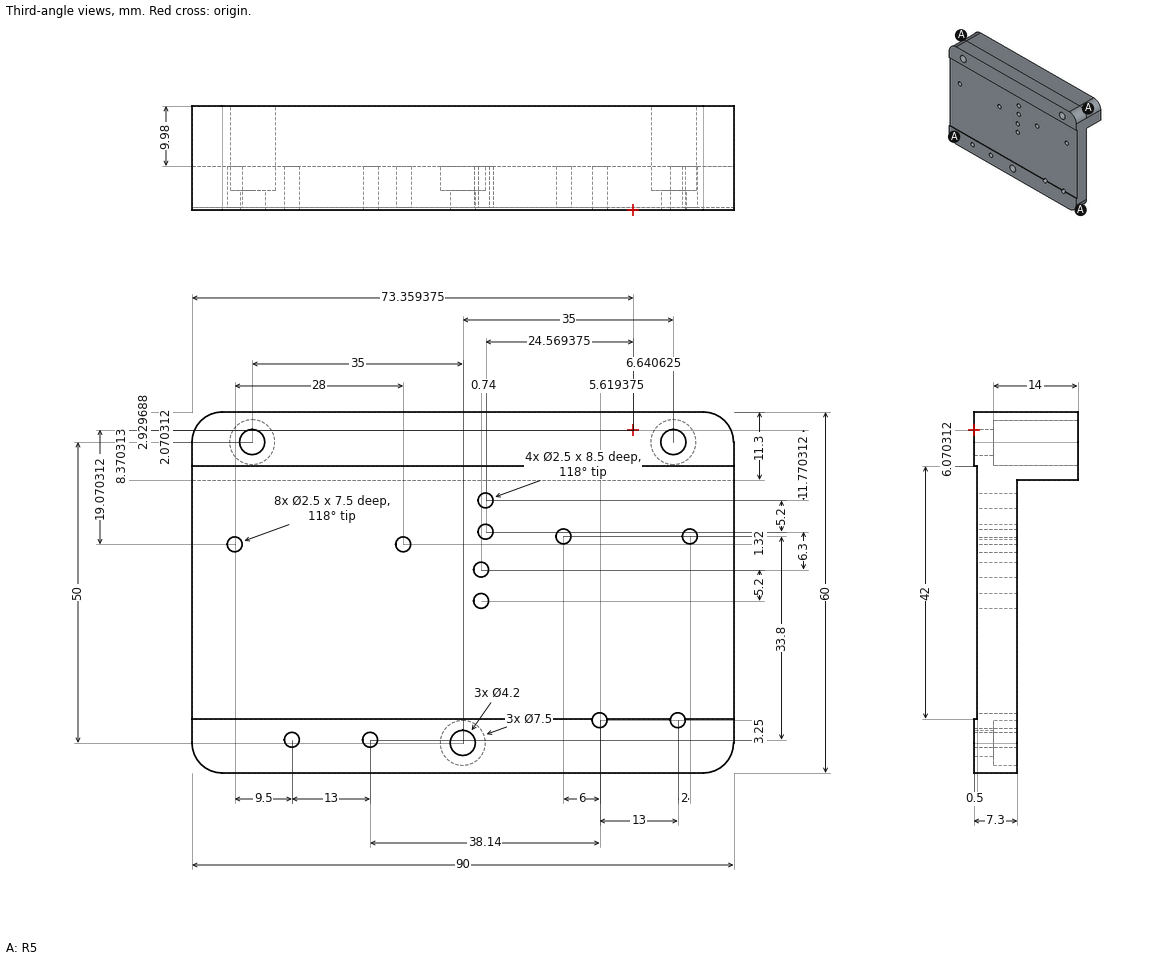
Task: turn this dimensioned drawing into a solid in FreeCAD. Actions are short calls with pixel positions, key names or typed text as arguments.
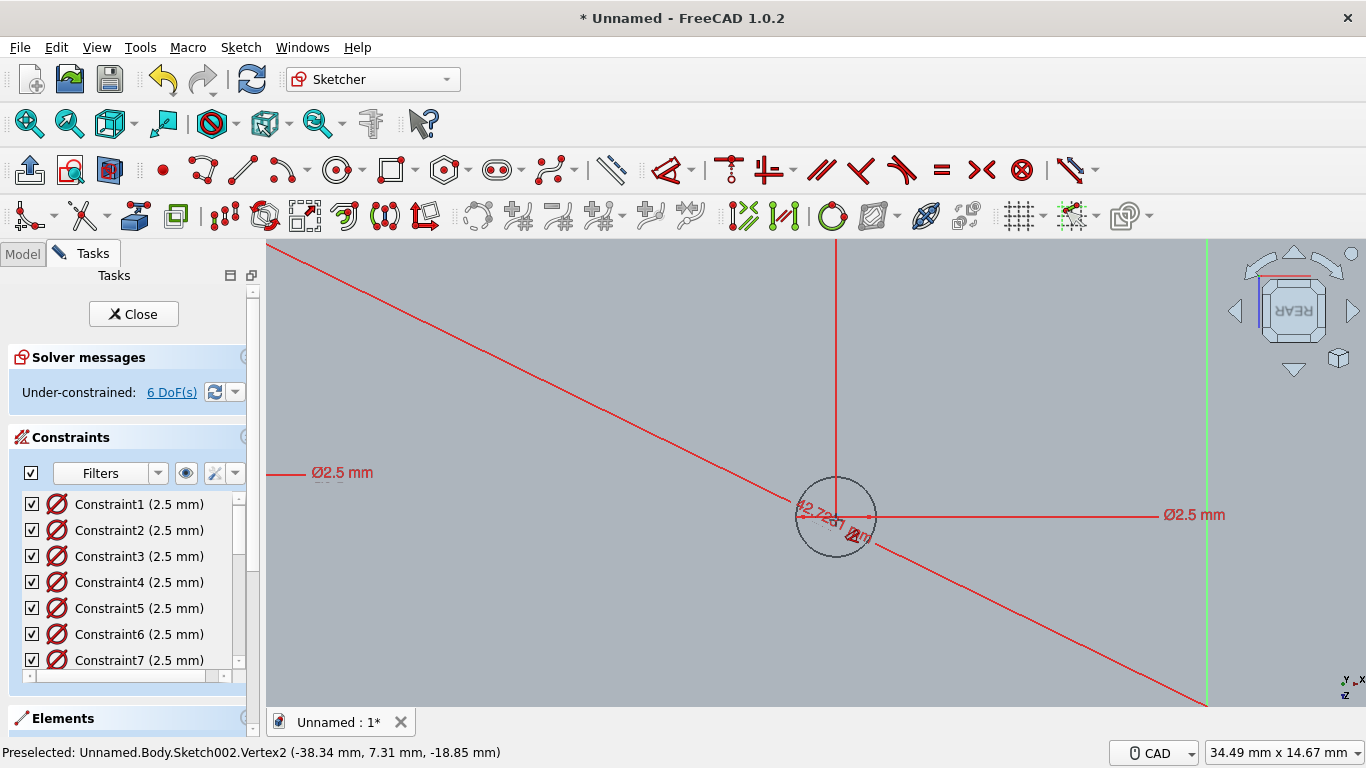
click(836, 517)
click(894, 496)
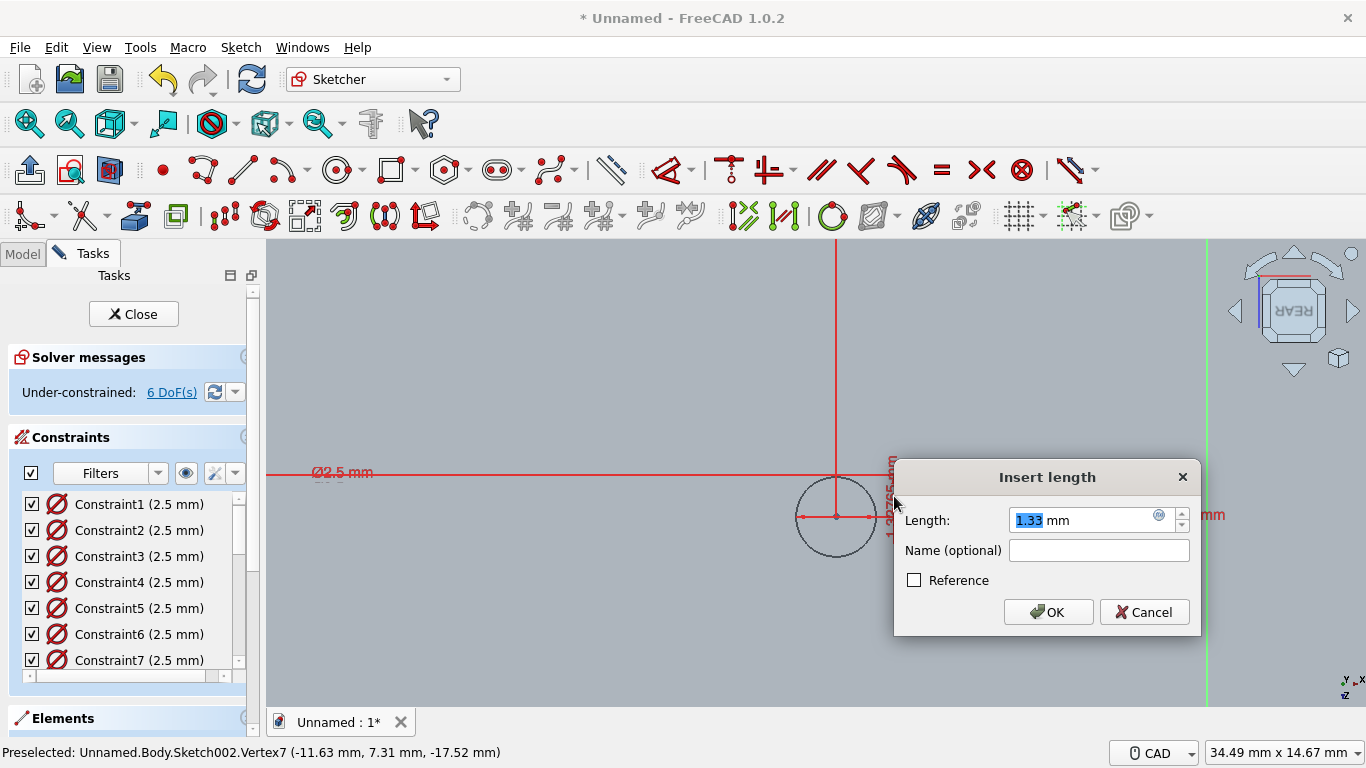
text(1.32)
key(Return)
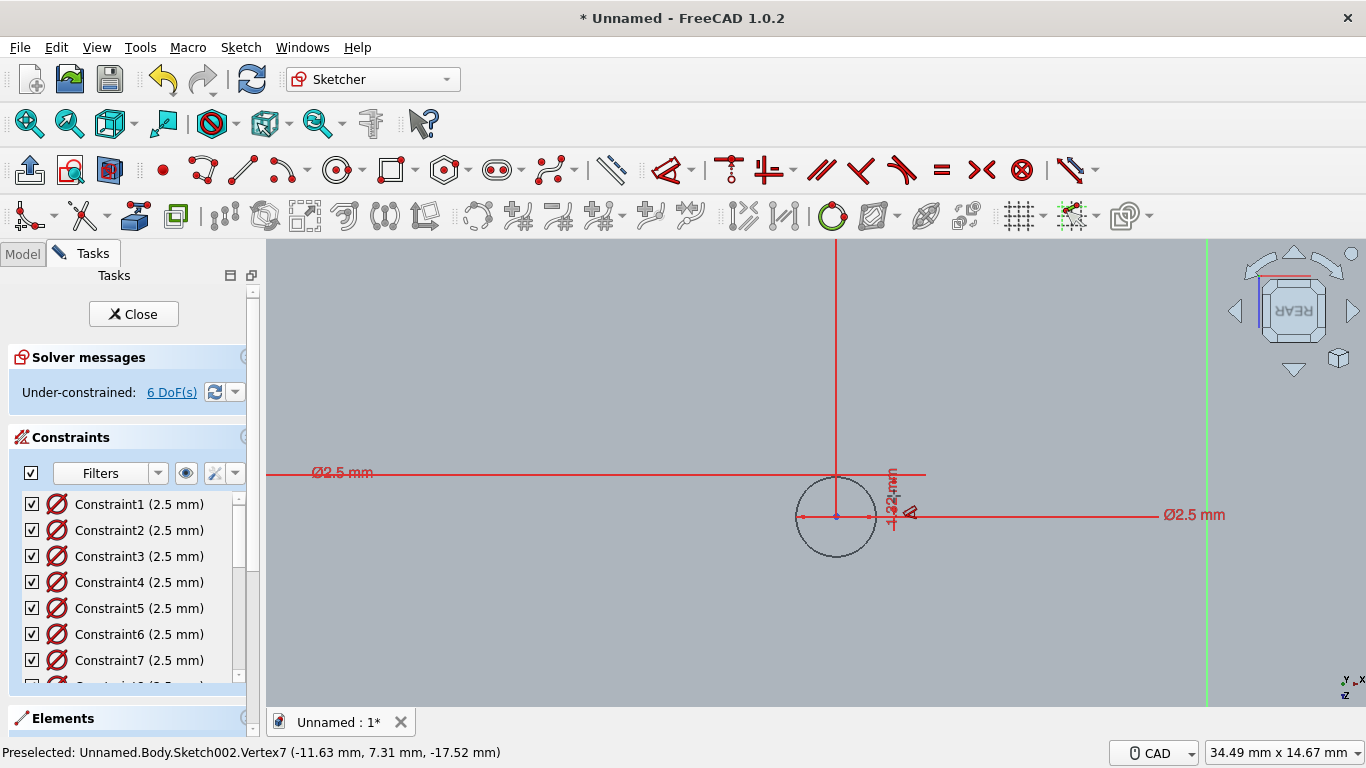
scroll(836, 520, down, 9)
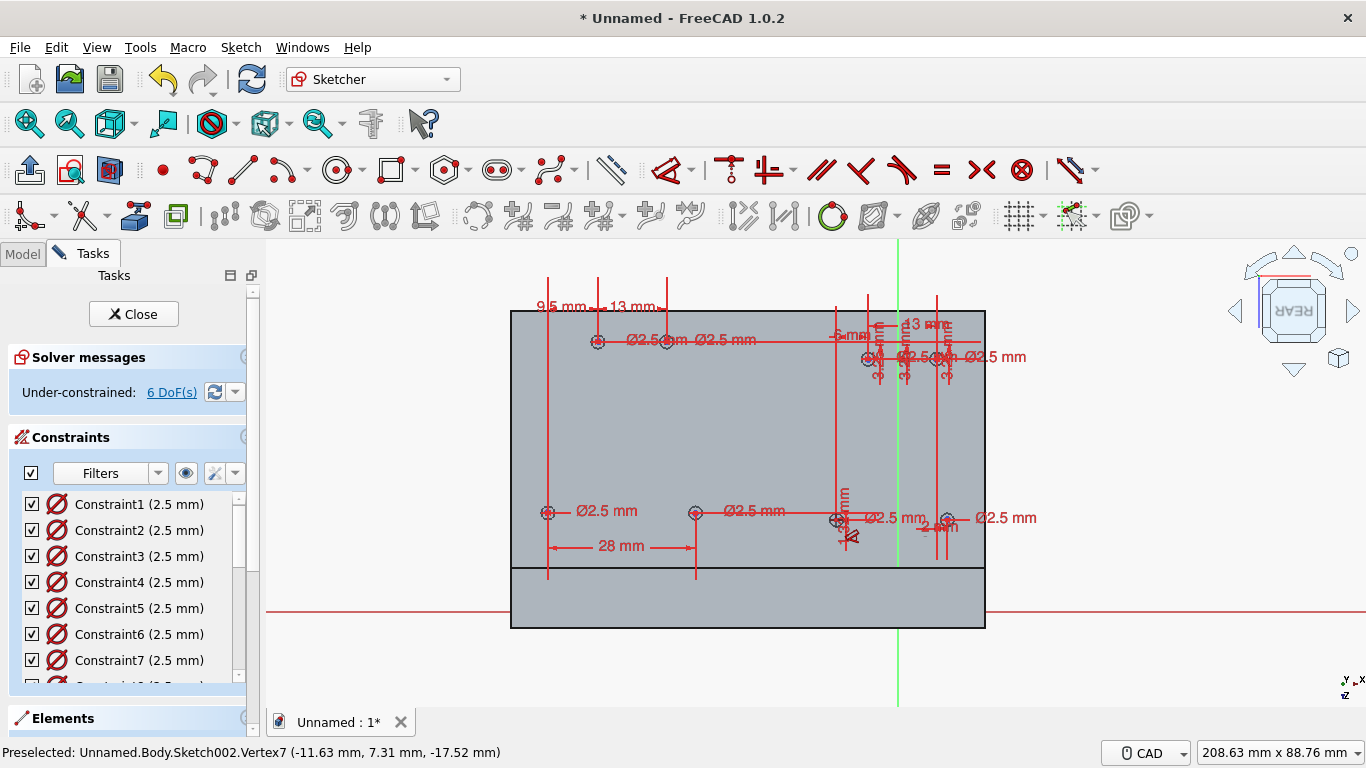
click(667, 342)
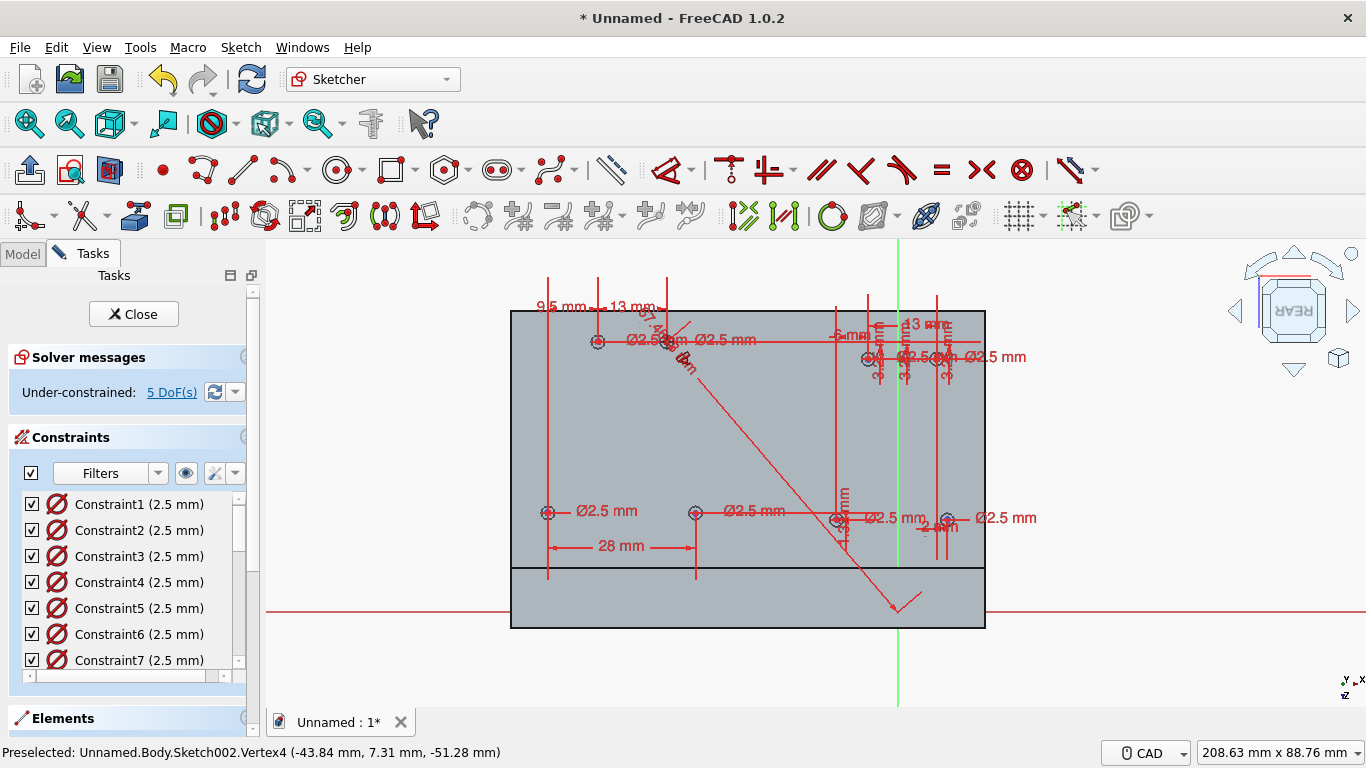
click(836, 520)
click(870, 431)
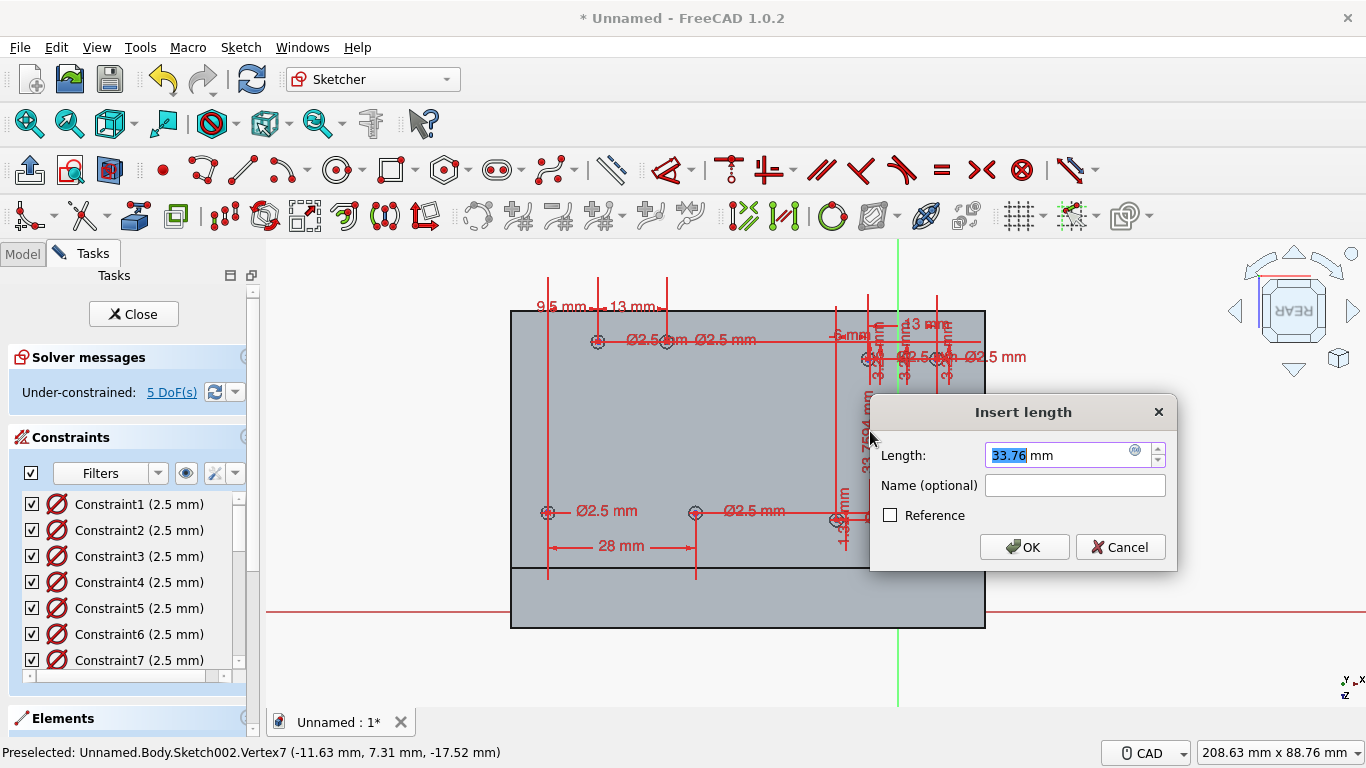
text(33.8)
key(Return)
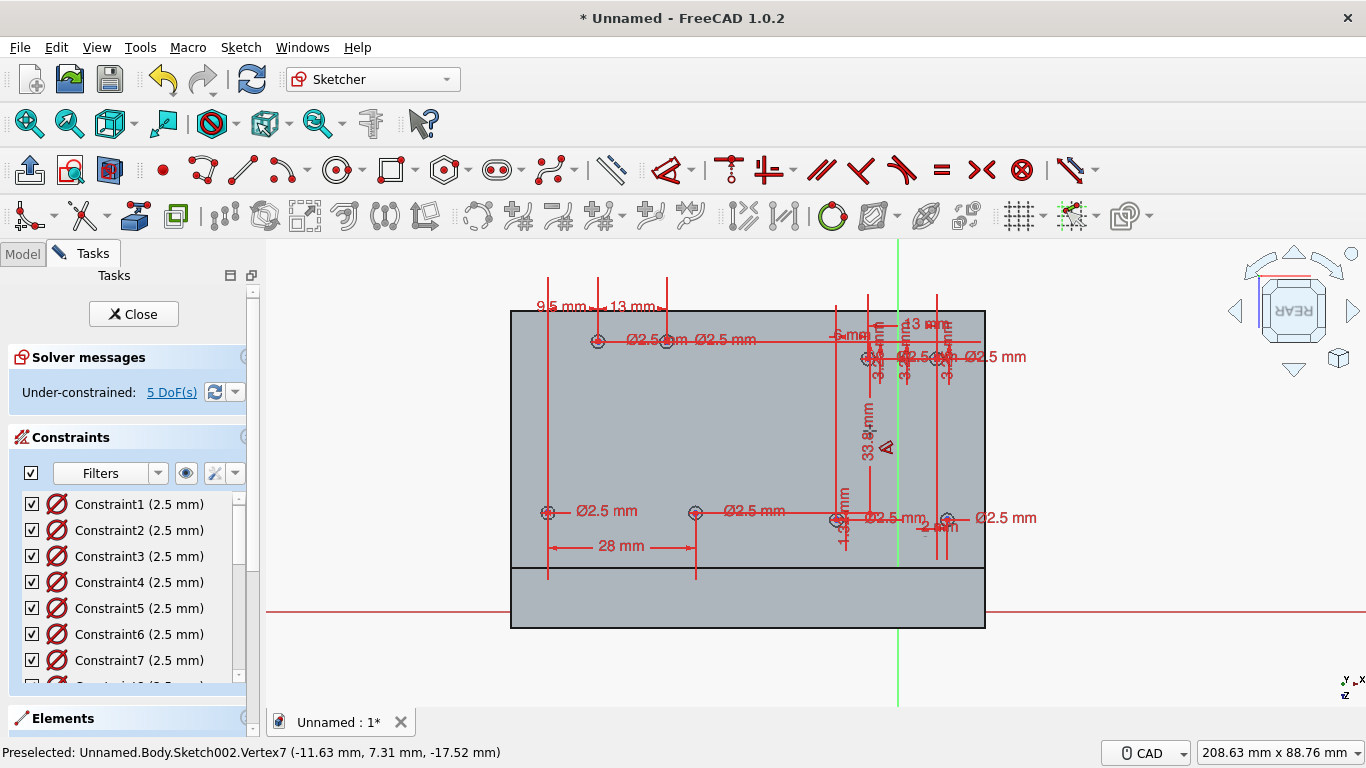
scroll(548, 513, up, 9)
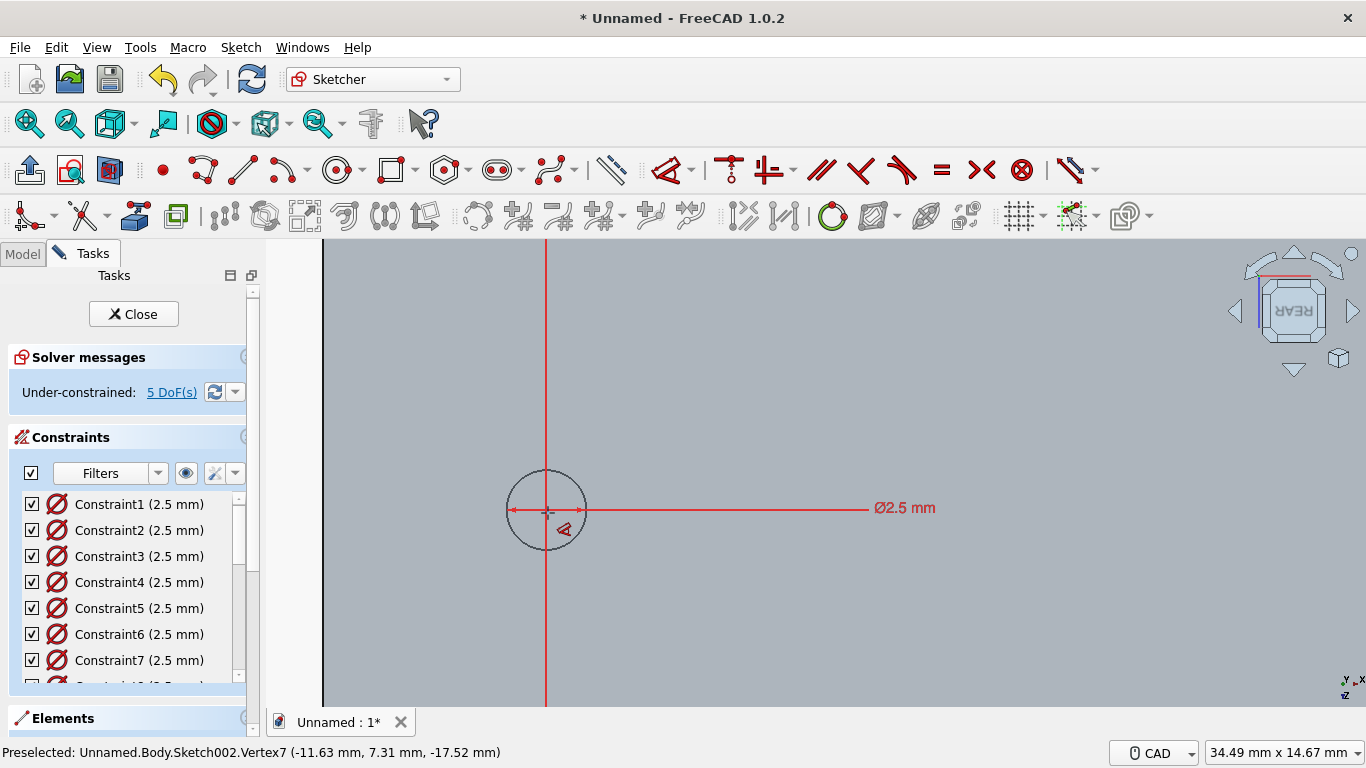
click(546, 510)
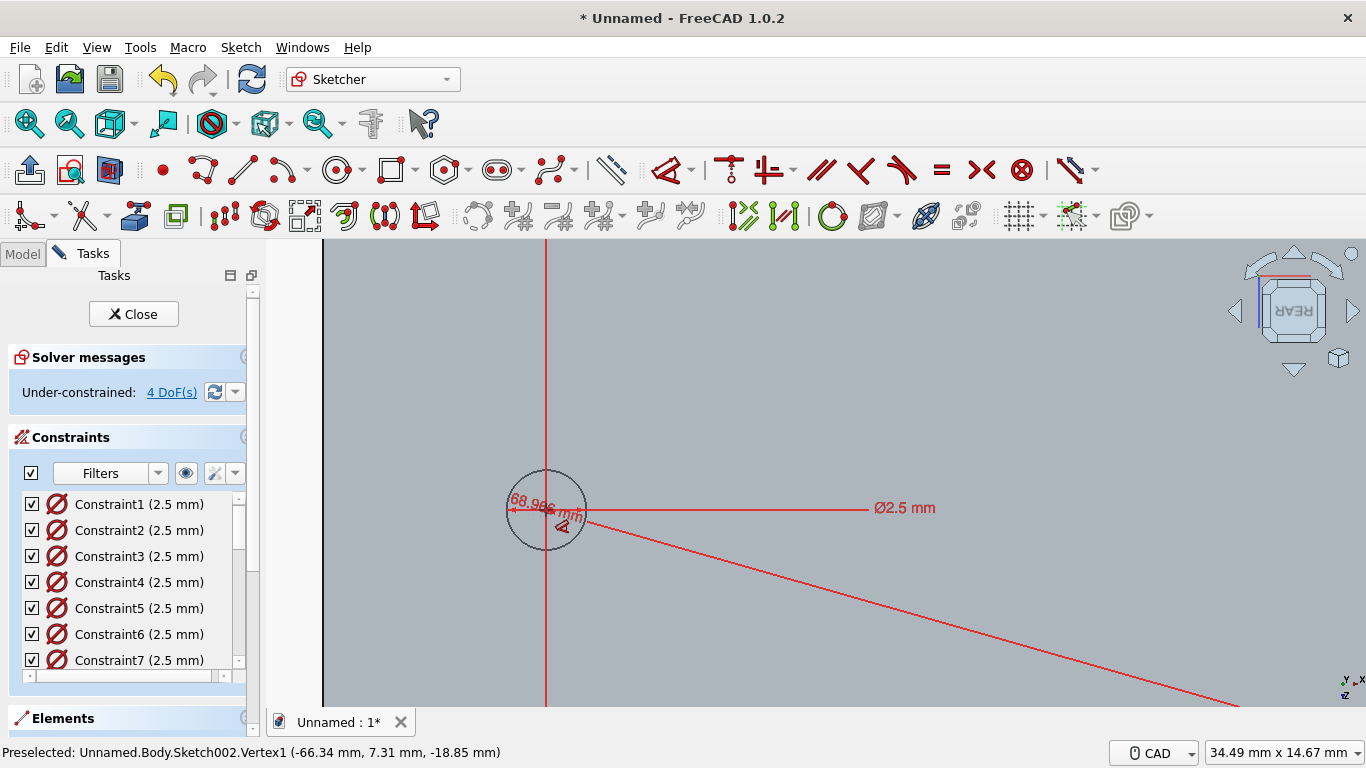
scroll(548, 513, down, 9)